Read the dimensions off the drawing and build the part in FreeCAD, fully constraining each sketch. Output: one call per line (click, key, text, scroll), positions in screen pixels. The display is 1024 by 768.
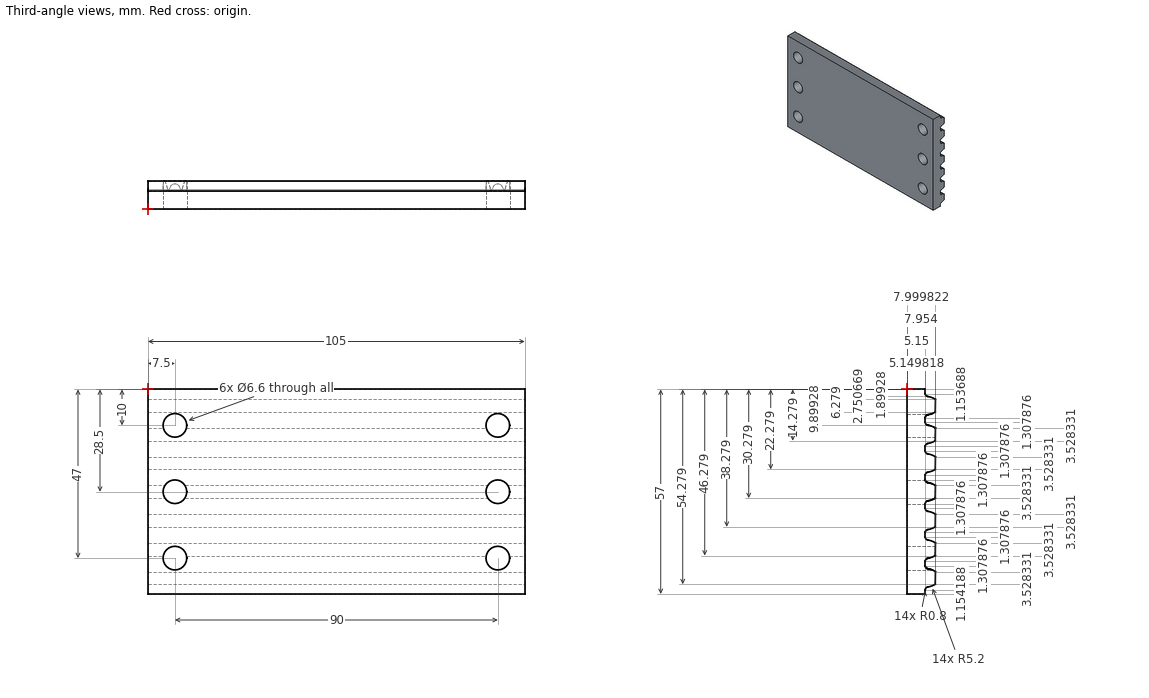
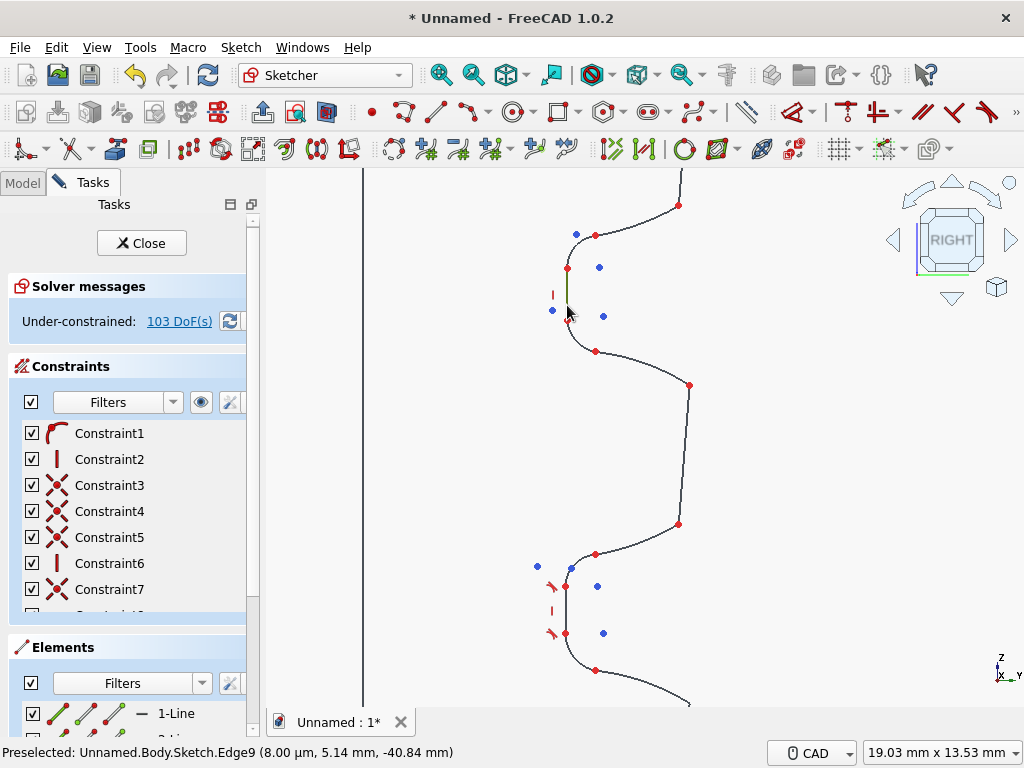
click(571, 333)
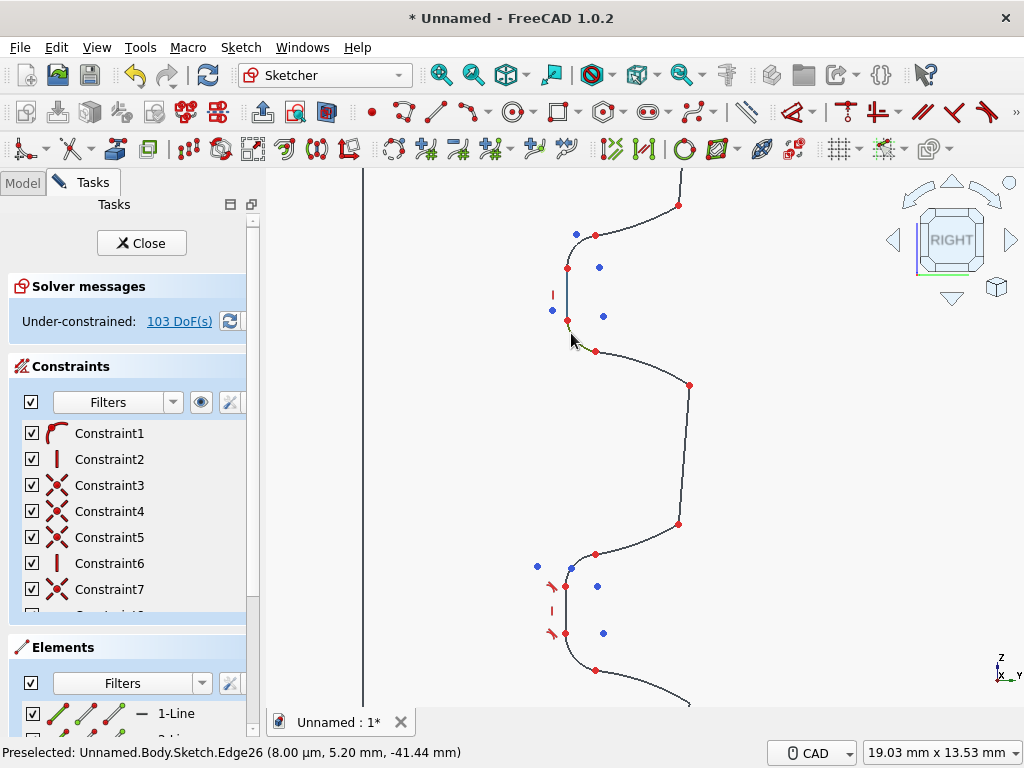
click(988, 112)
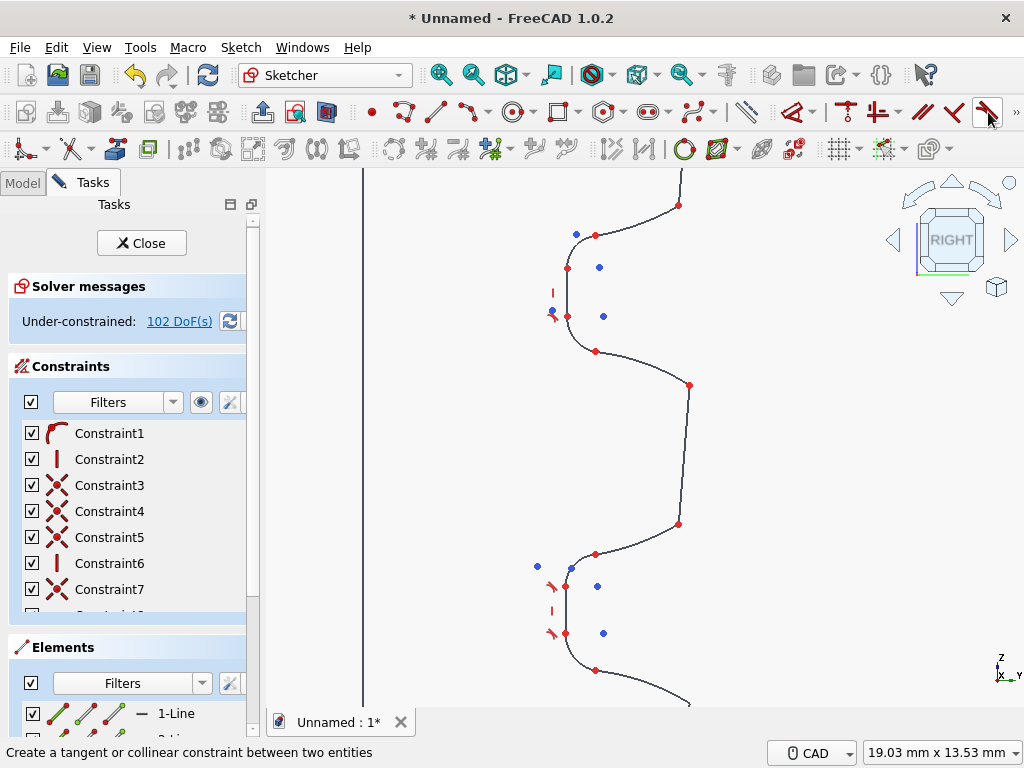
click(567, 302)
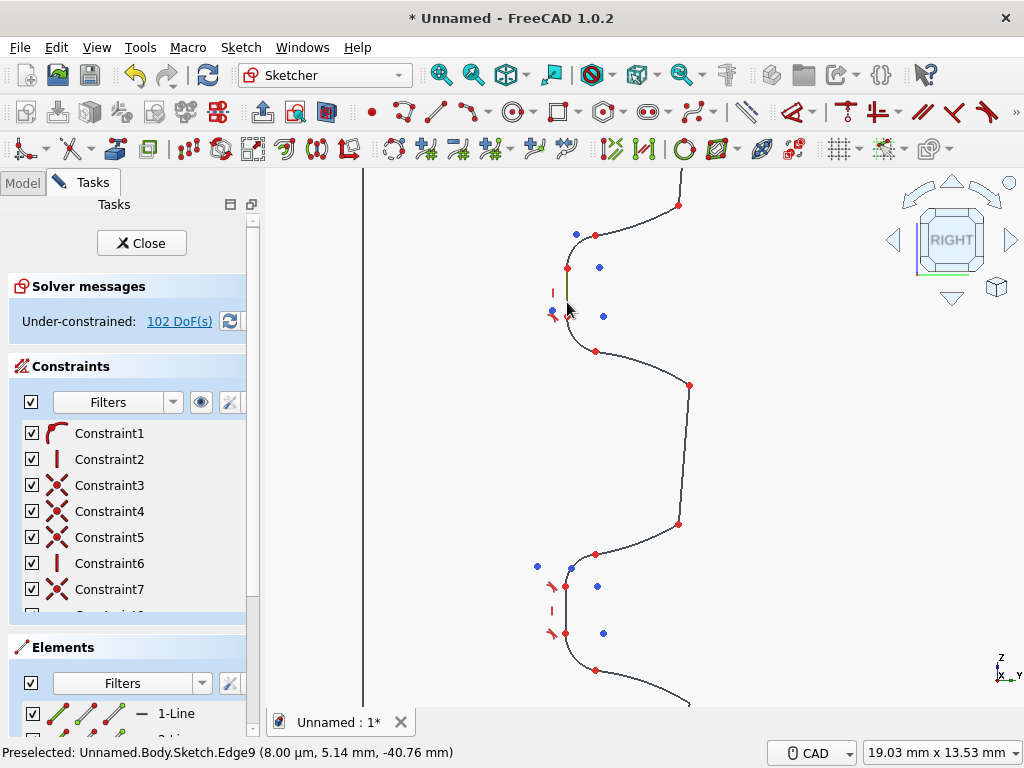
click(582, 241)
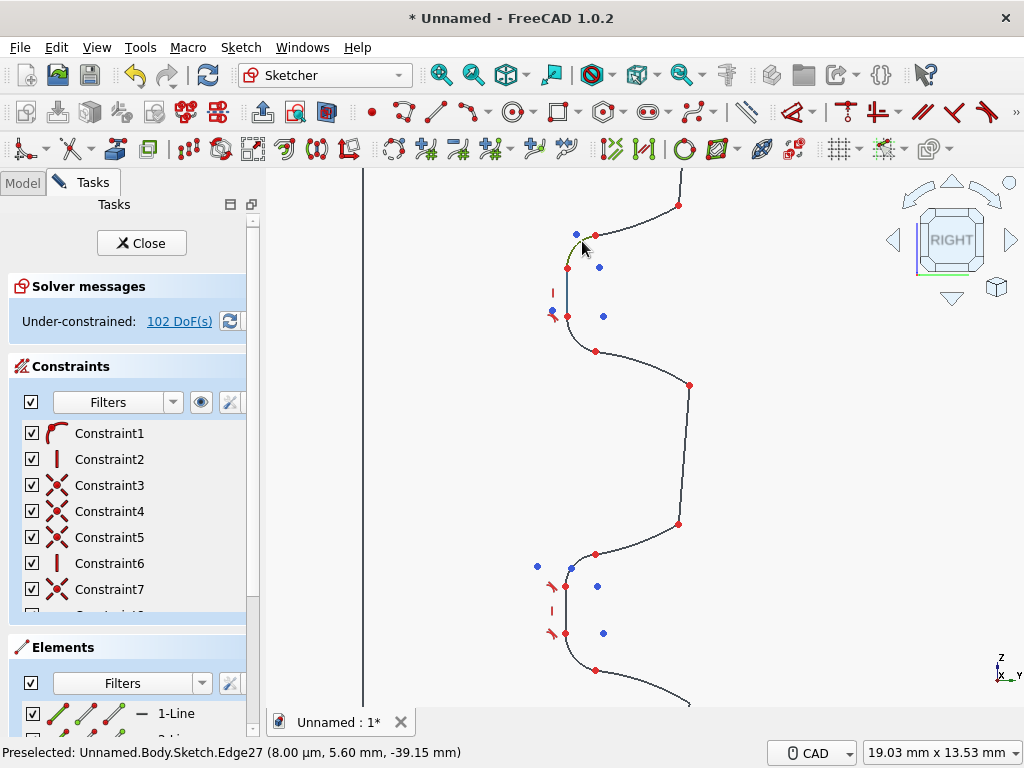
click(988, 112)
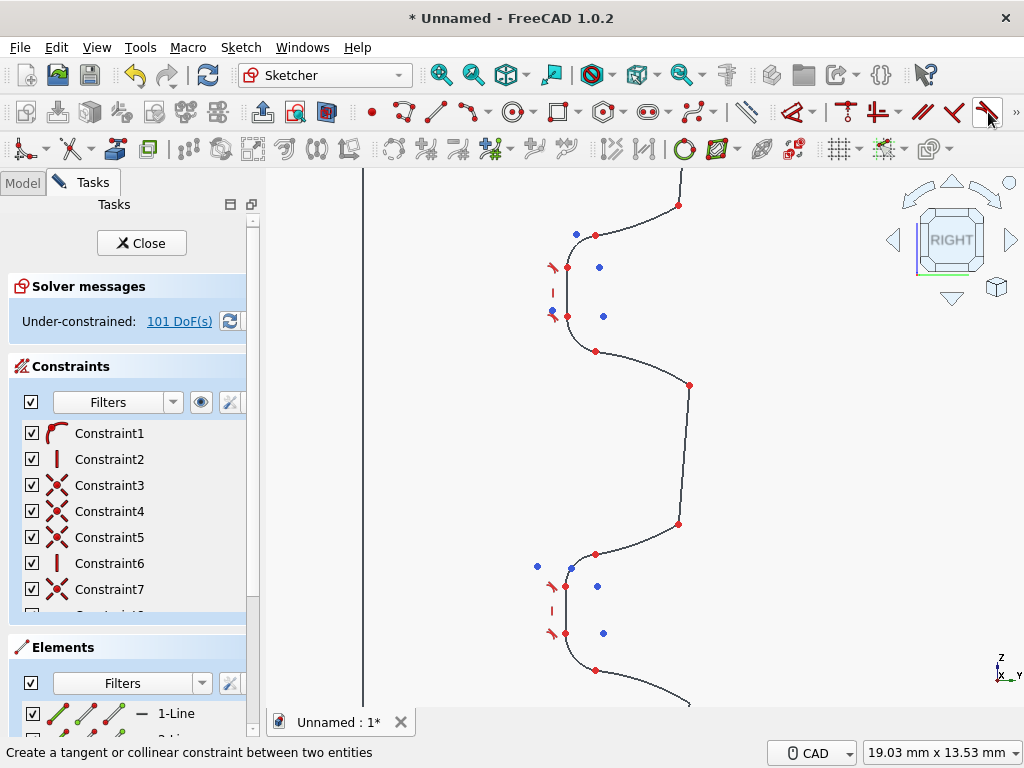
scroll(587, 561, down, 9)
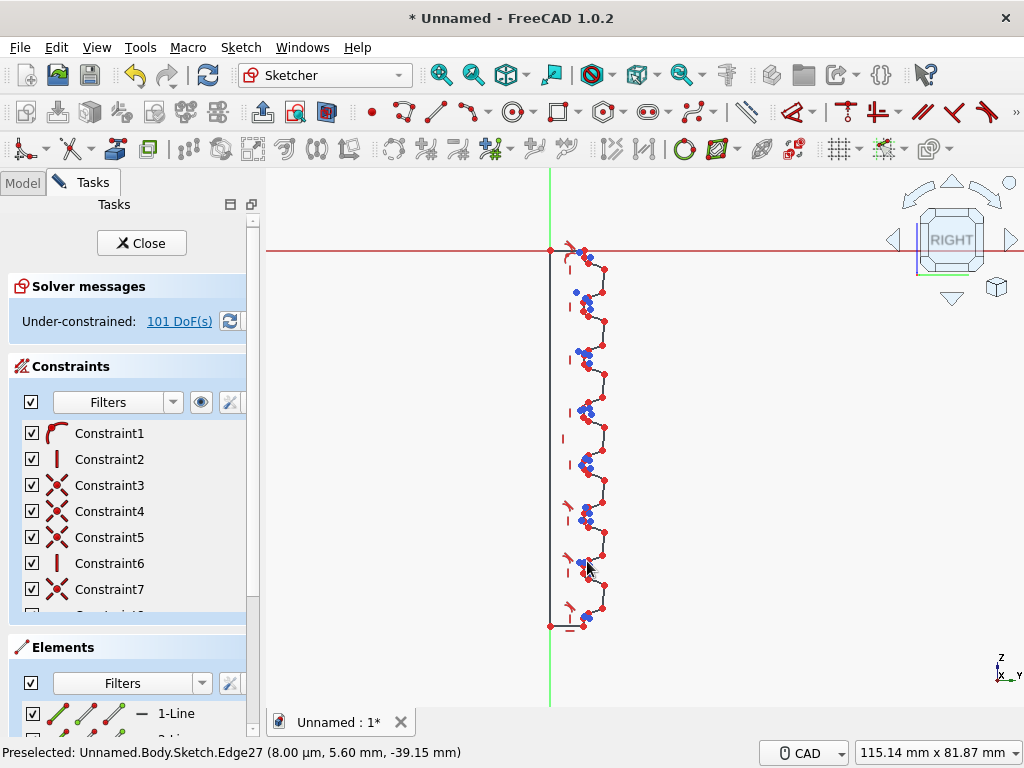
scroll(584, 467, up, 9)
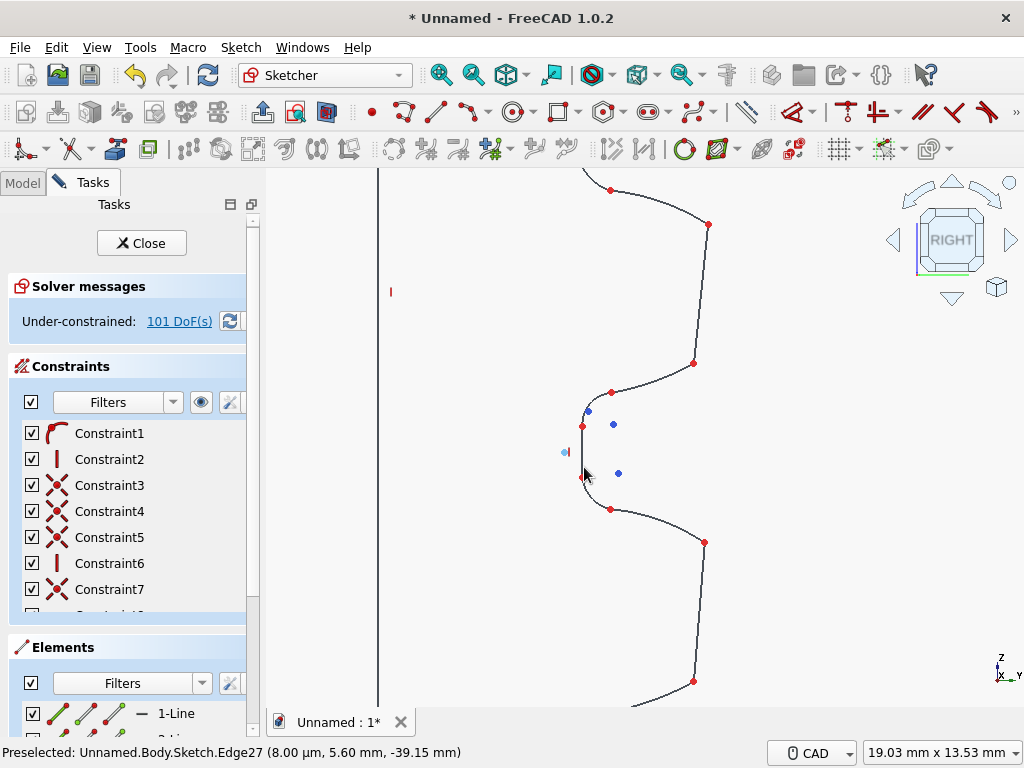
click(582, 462)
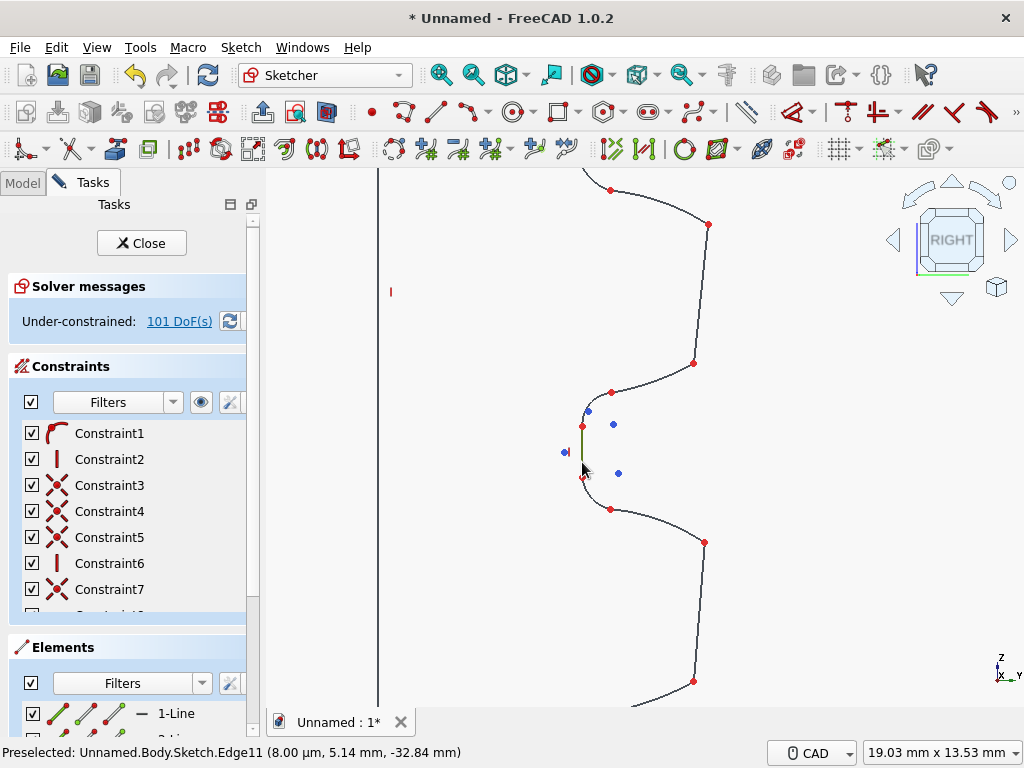
click(586, 491)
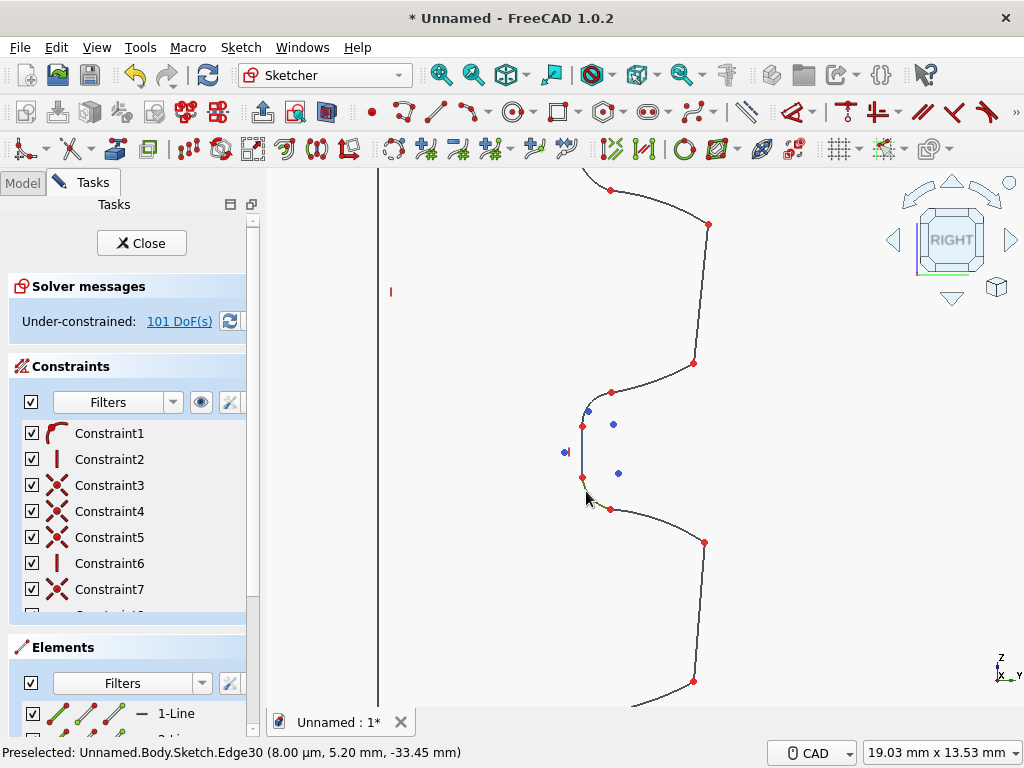
click(988, 112)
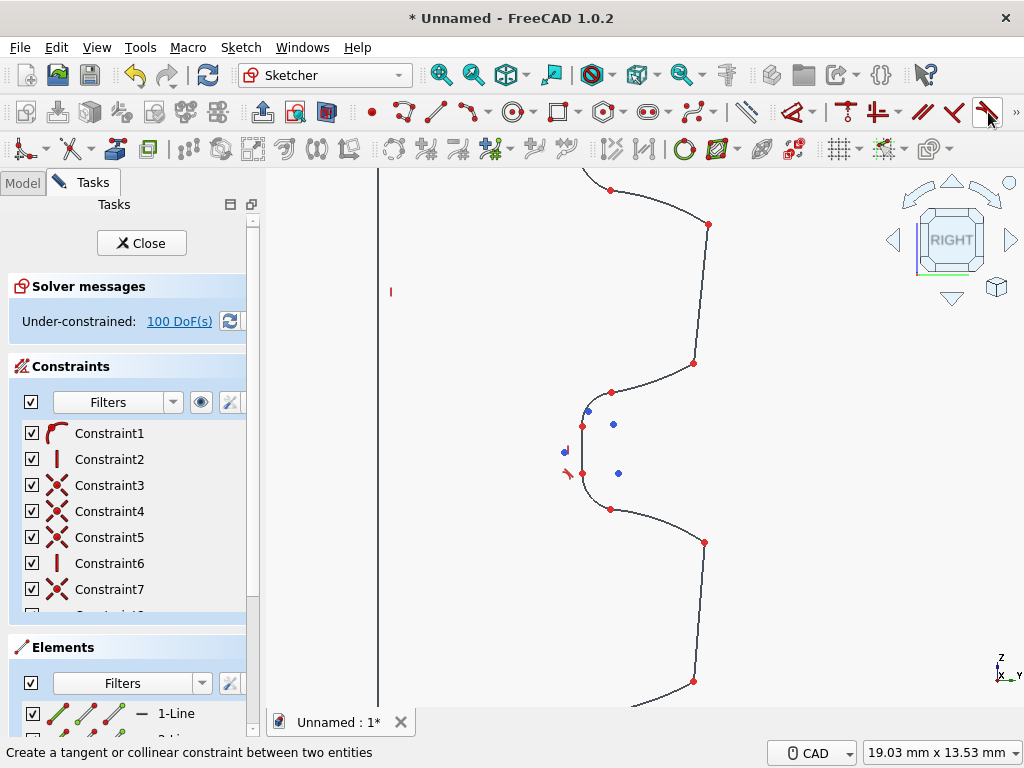
click(582, 459)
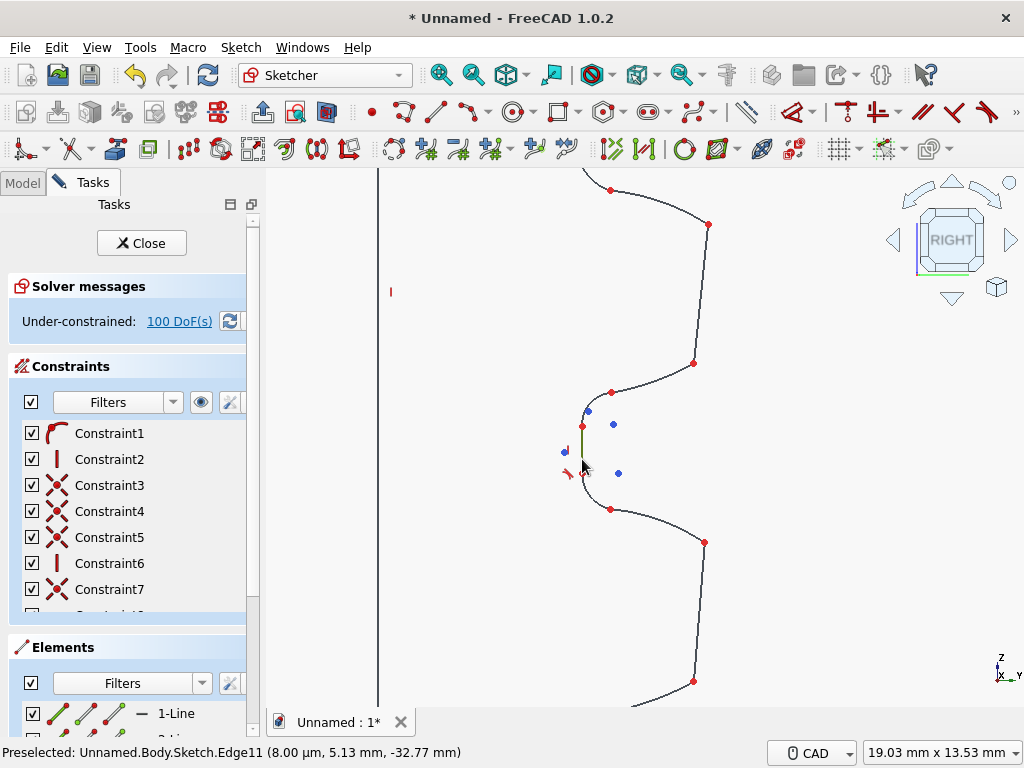
click(597, 397)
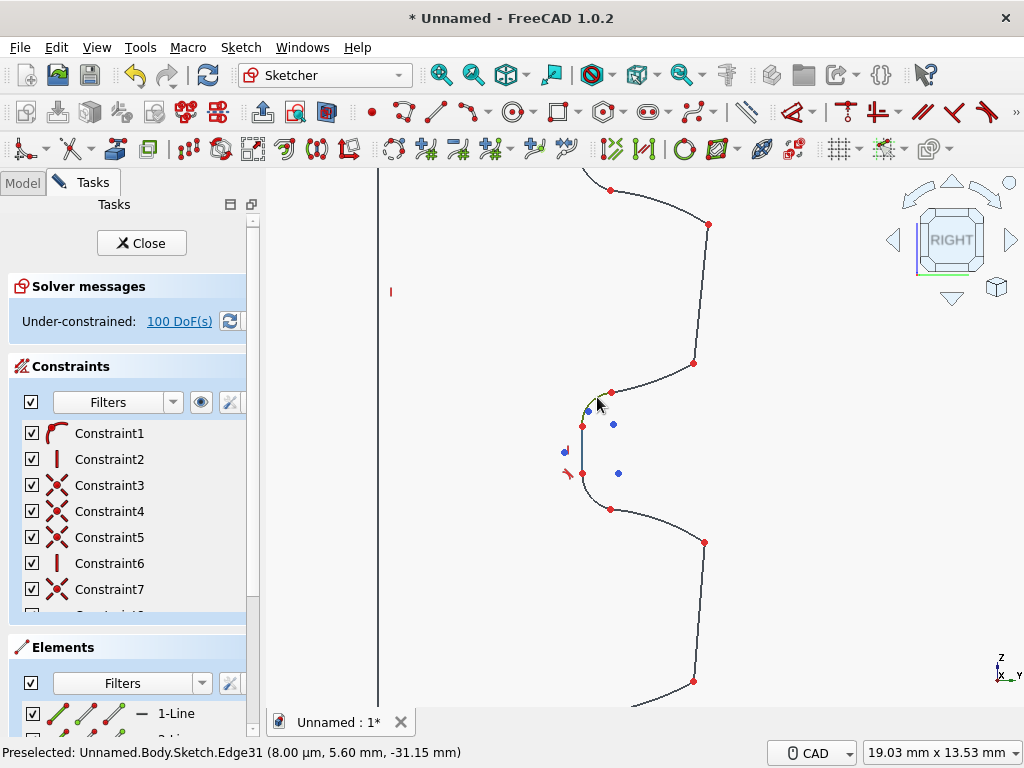
click(988, 112)